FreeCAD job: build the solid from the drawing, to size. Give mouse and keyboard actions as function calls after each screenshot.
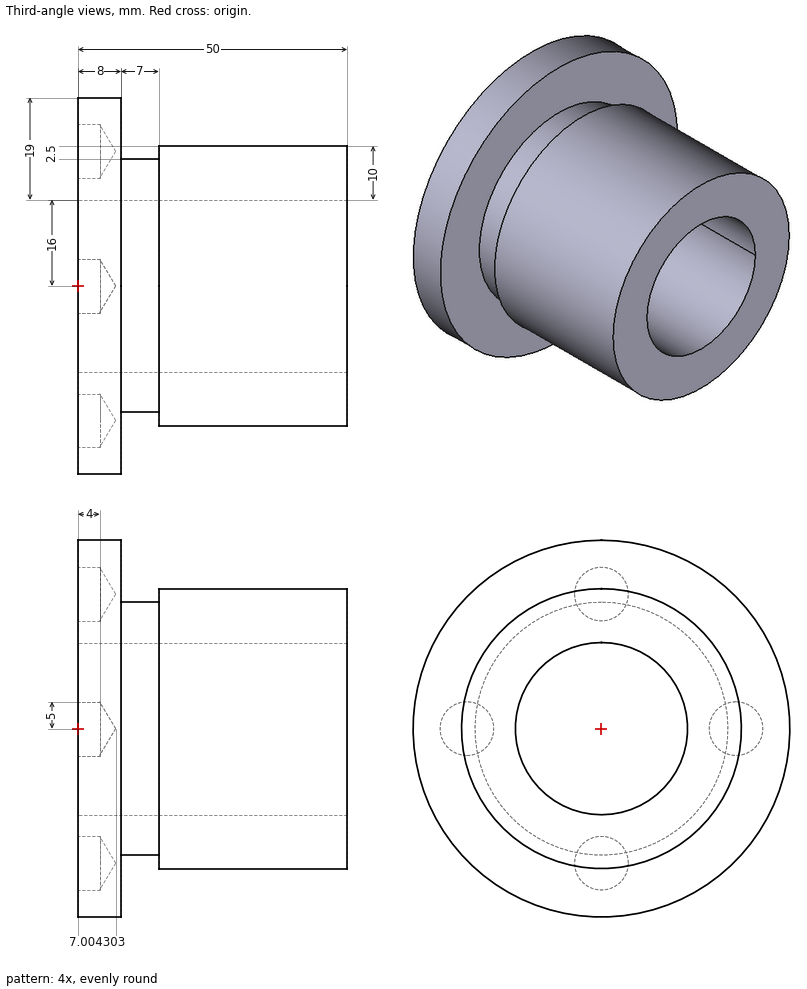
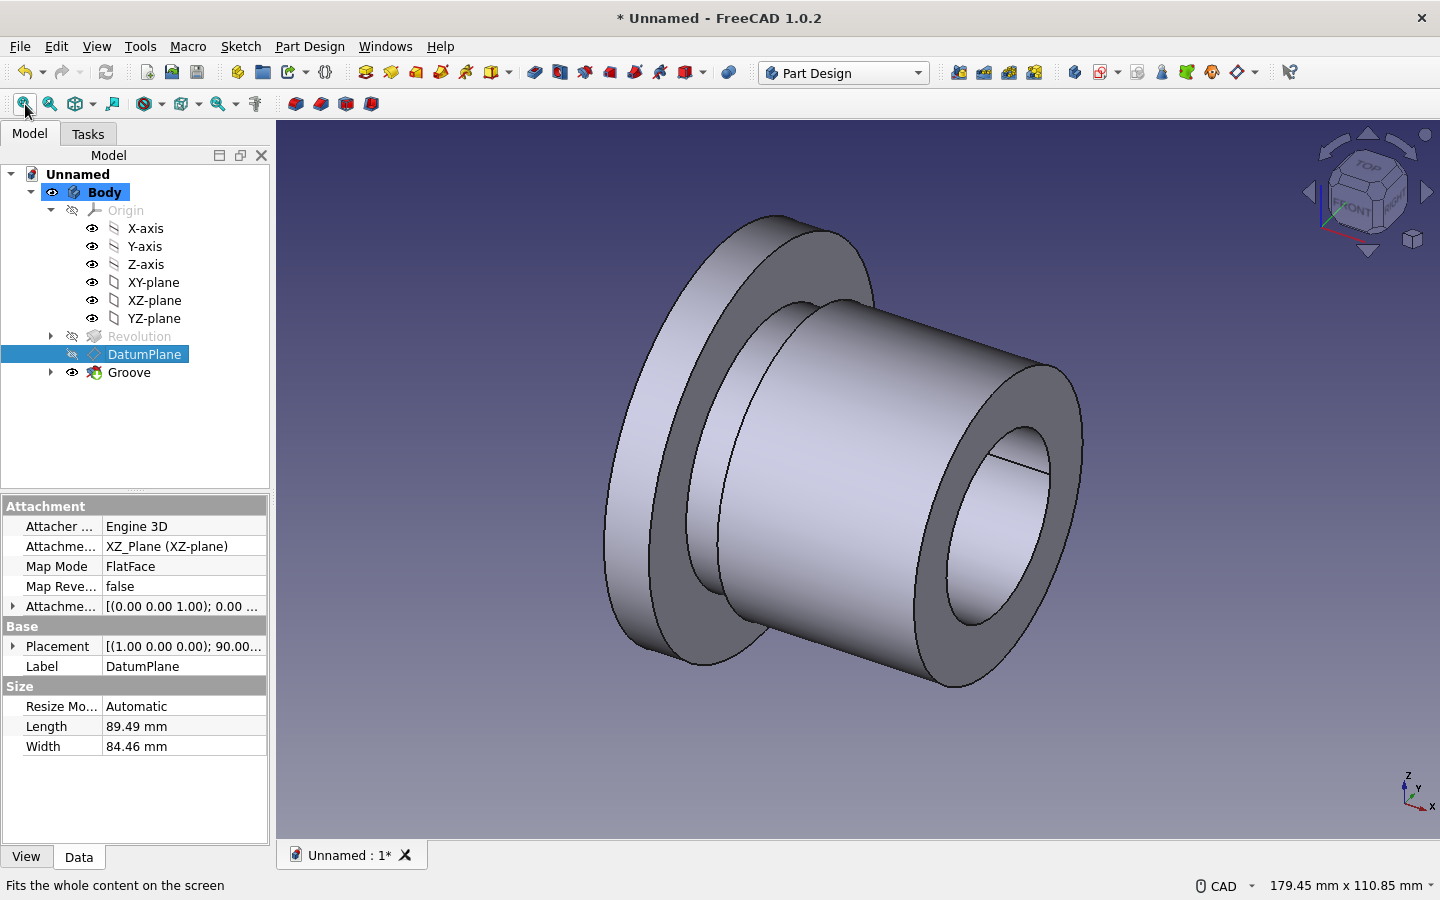
click(117, 372)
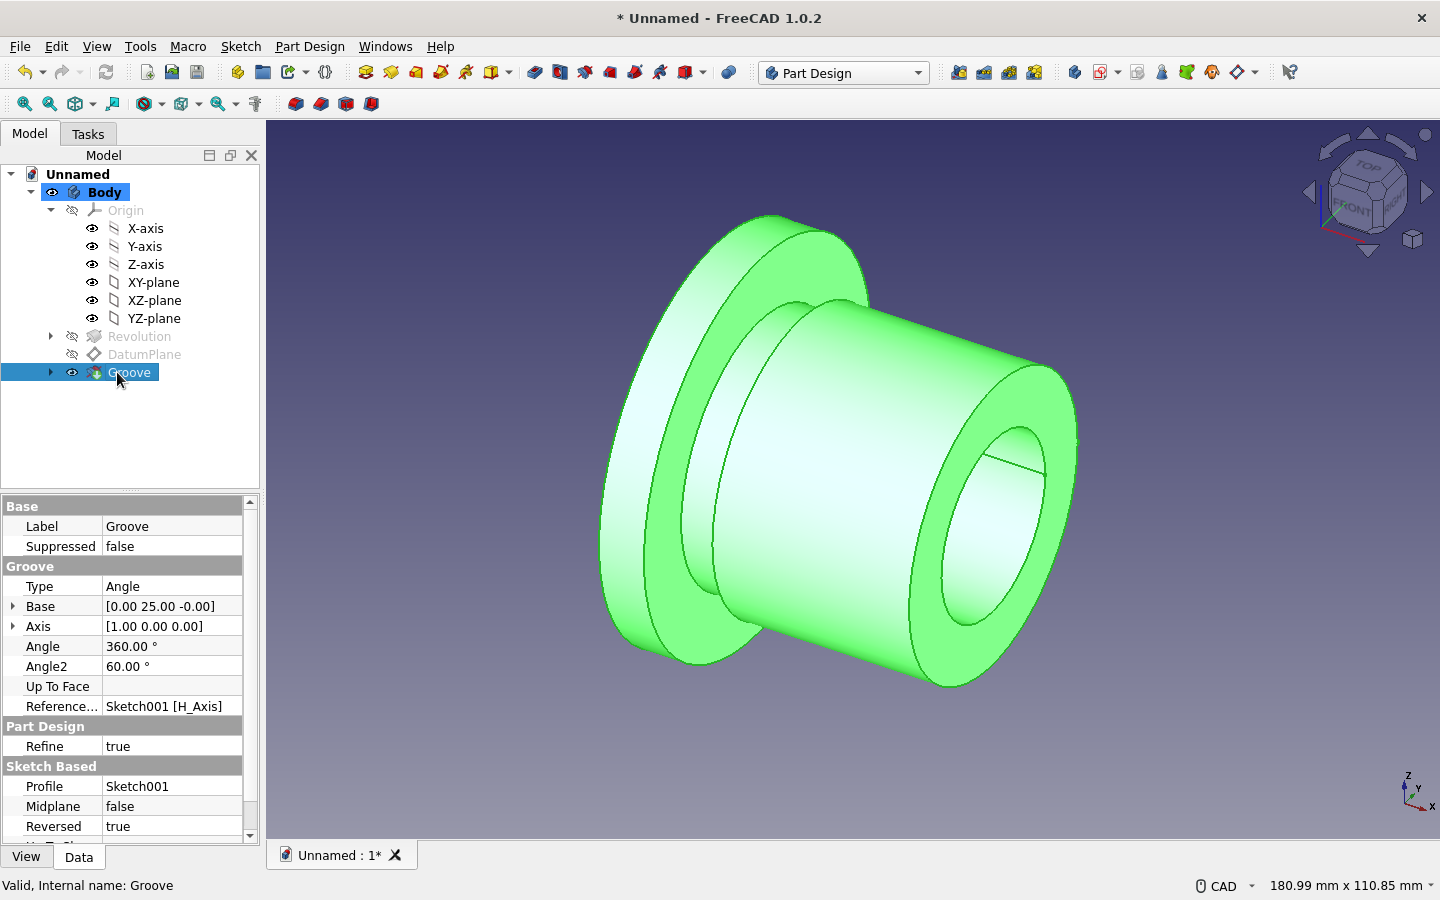
click(1009, 72)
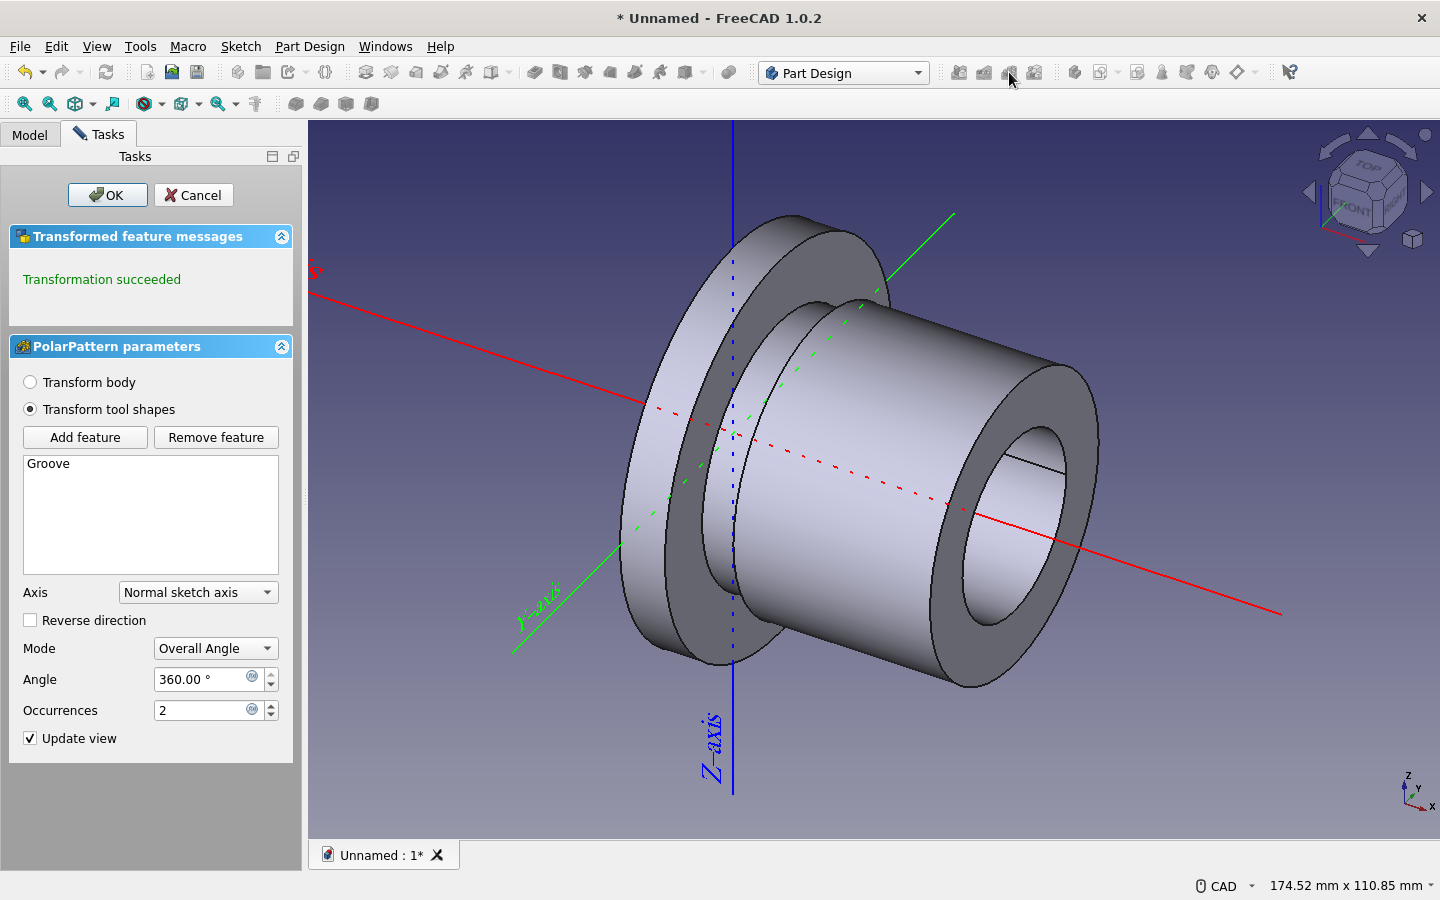
click(199, 592)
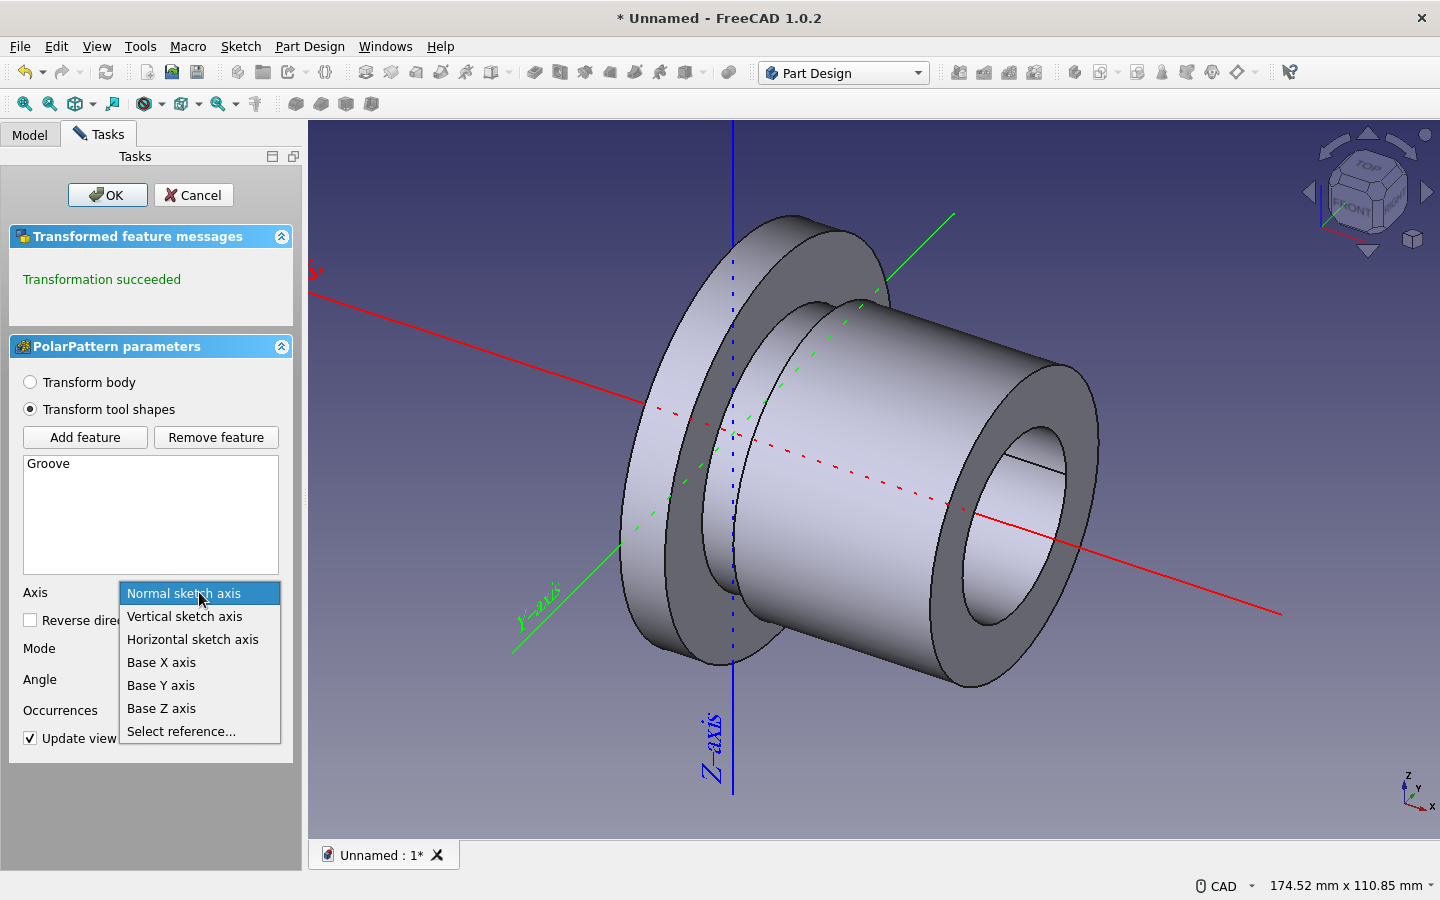
click(198, 662)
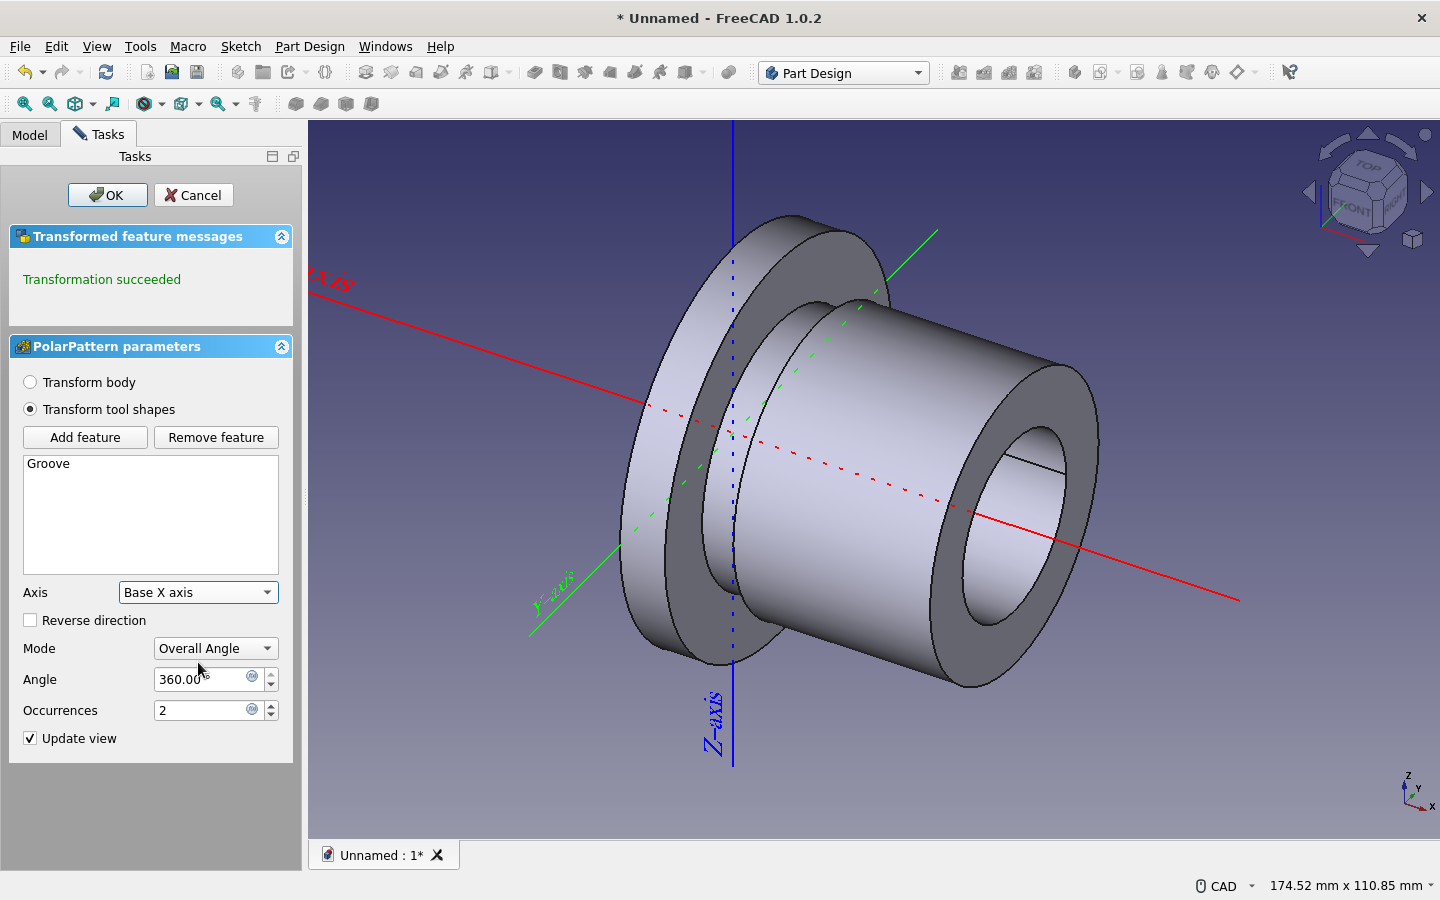
triple_click(210, 710)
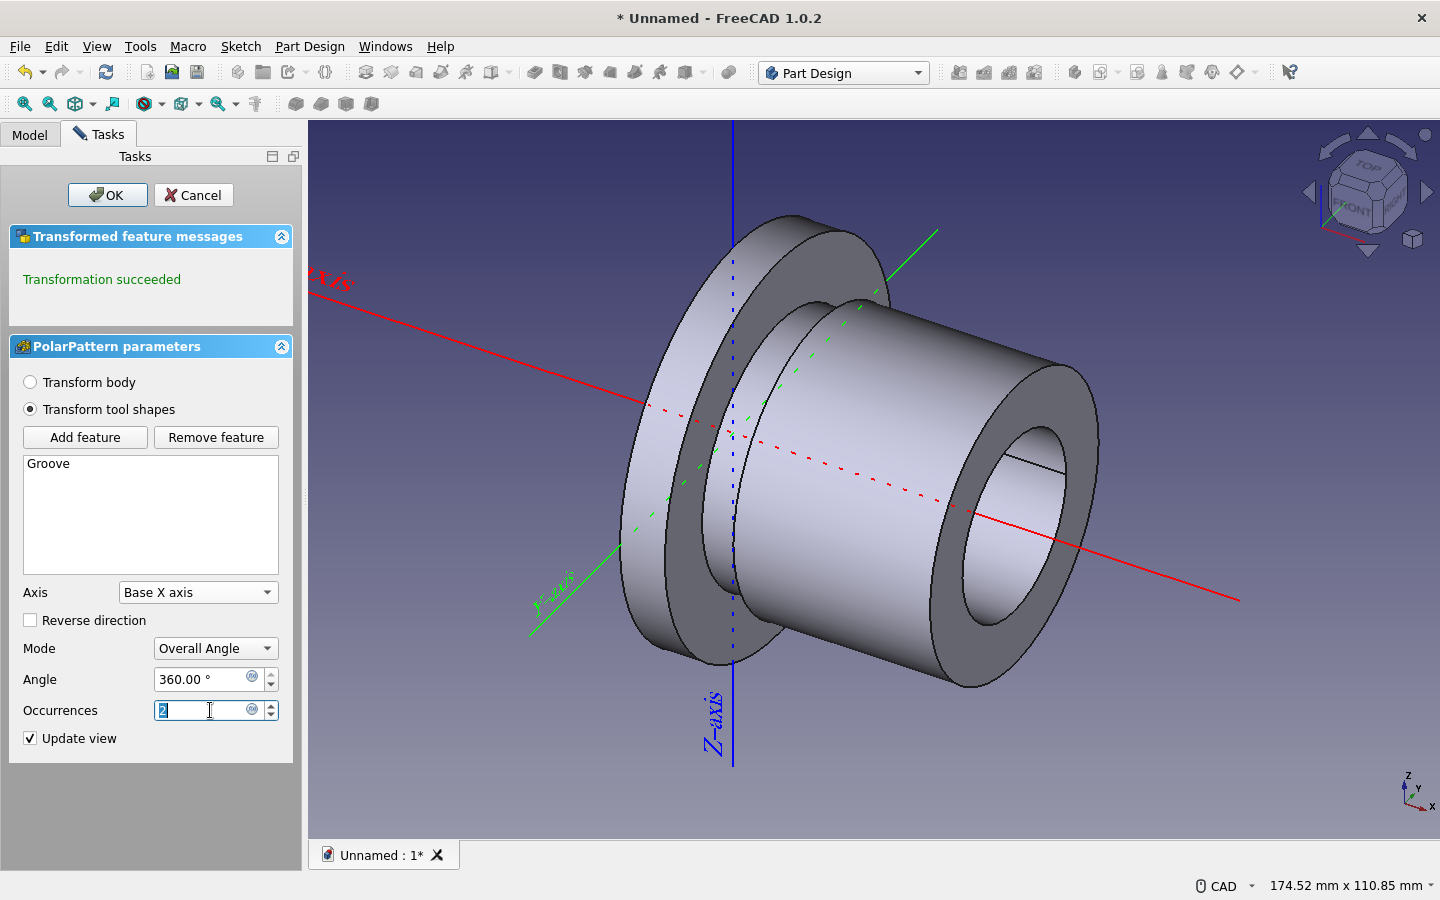
text(4)
key(Tab)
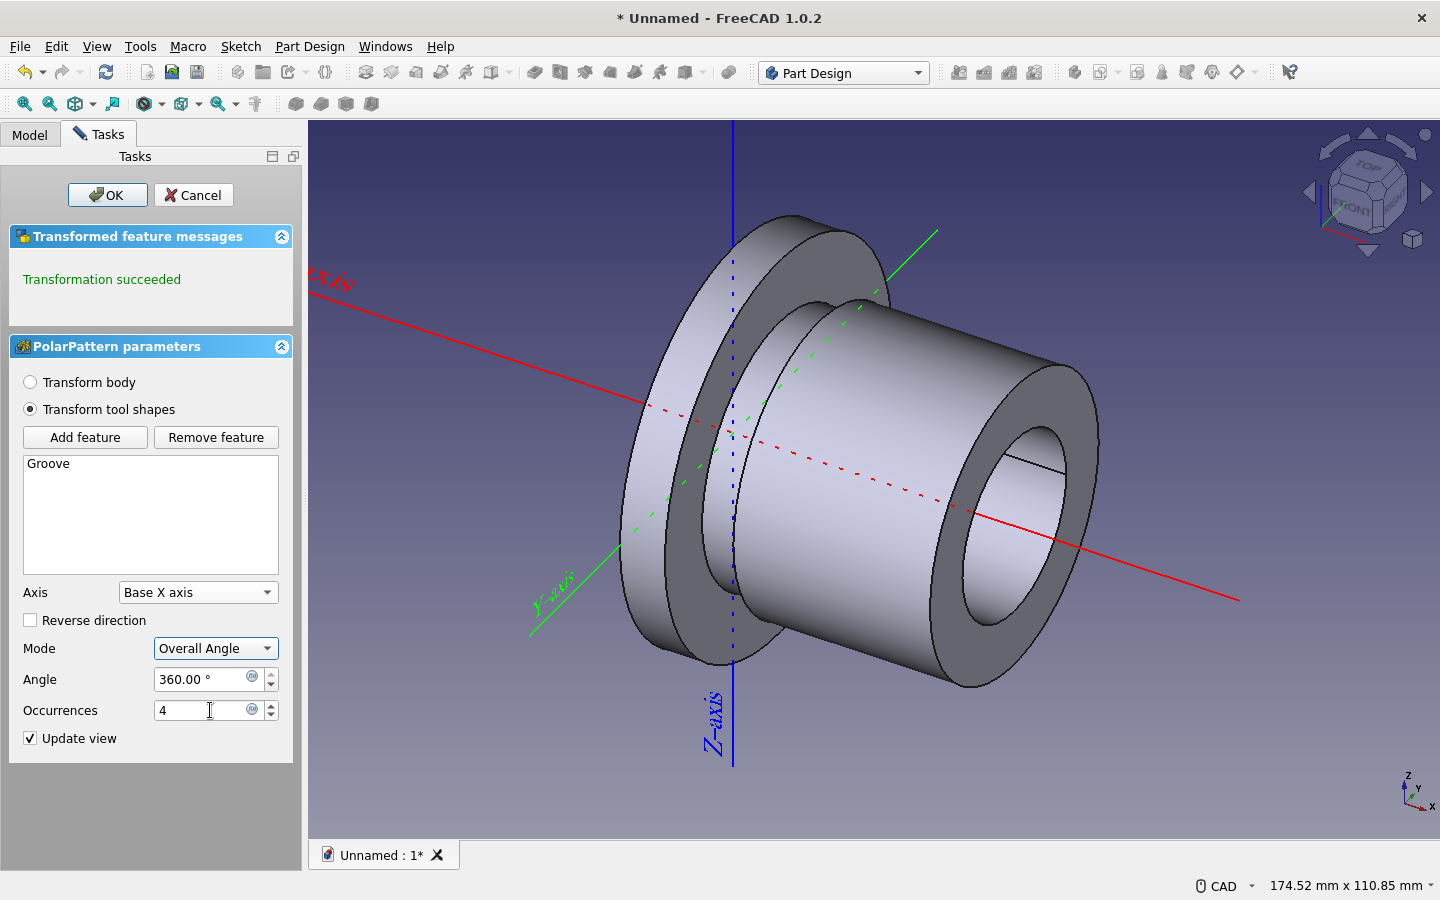
click(108, 195)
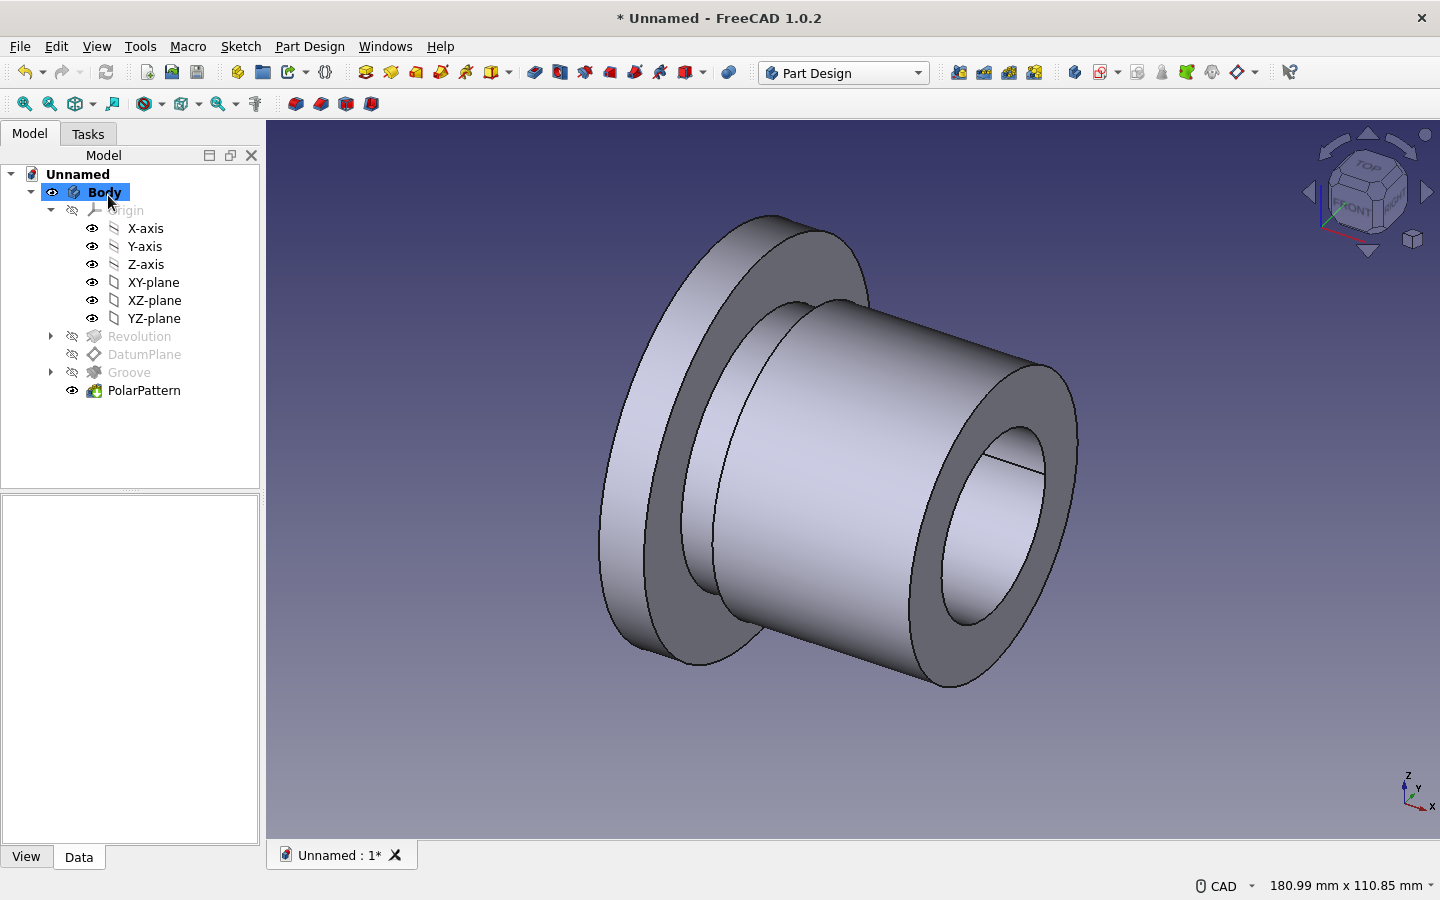
key(0)